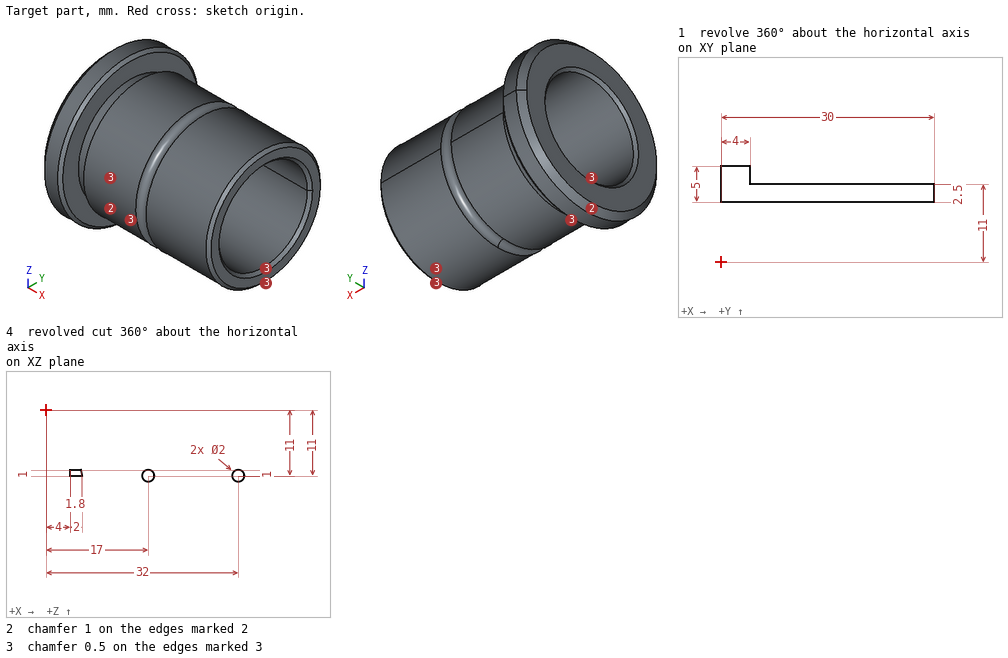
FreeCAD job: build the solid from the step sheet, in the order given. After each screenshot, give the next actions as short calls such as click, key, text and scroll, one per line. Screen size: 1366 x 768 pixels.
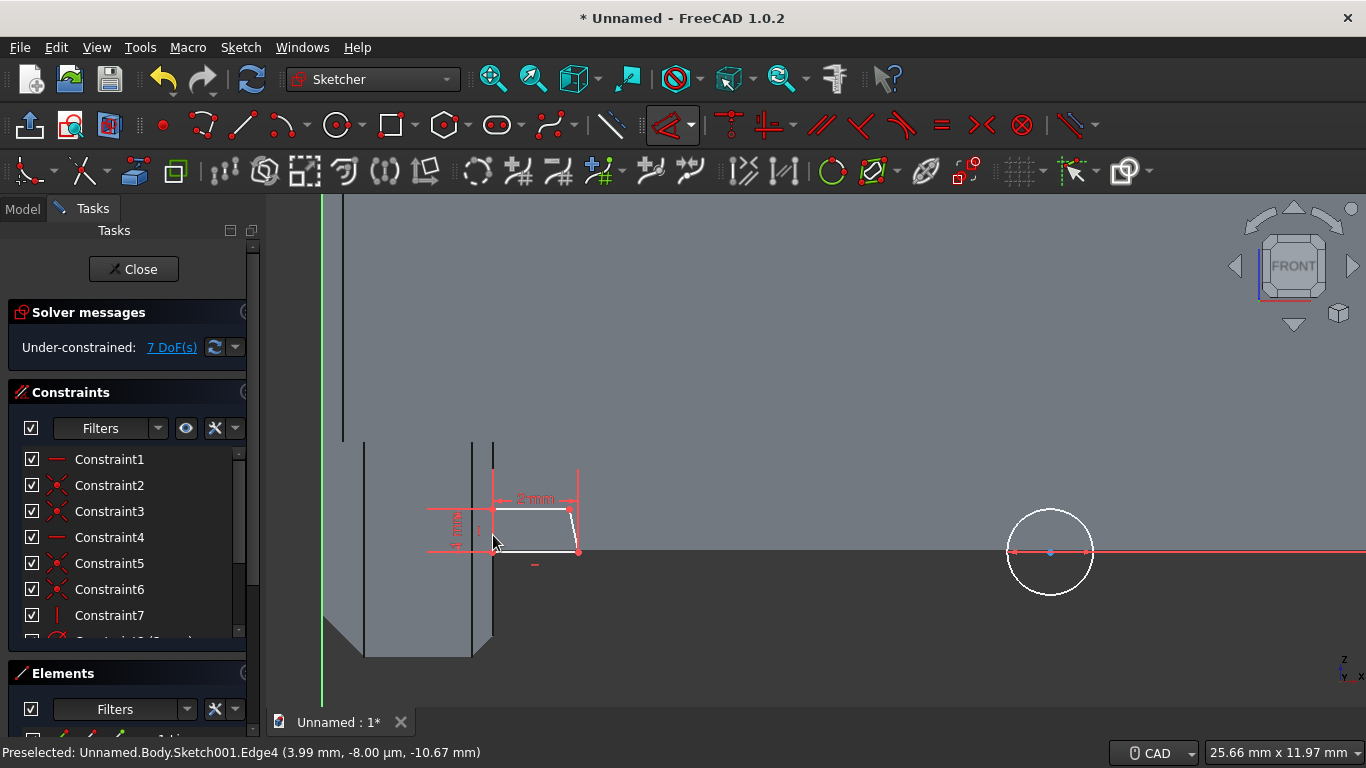
click(493, 509)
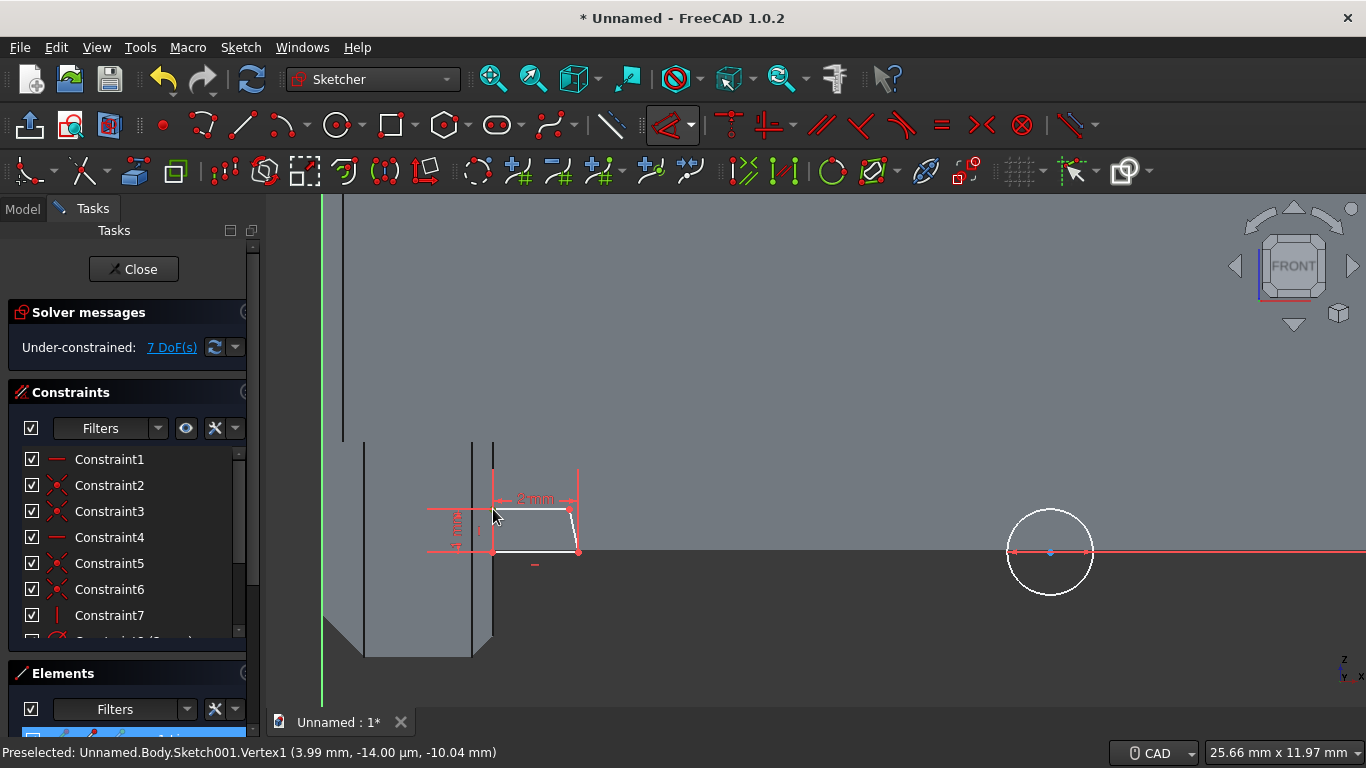
click(694, 126)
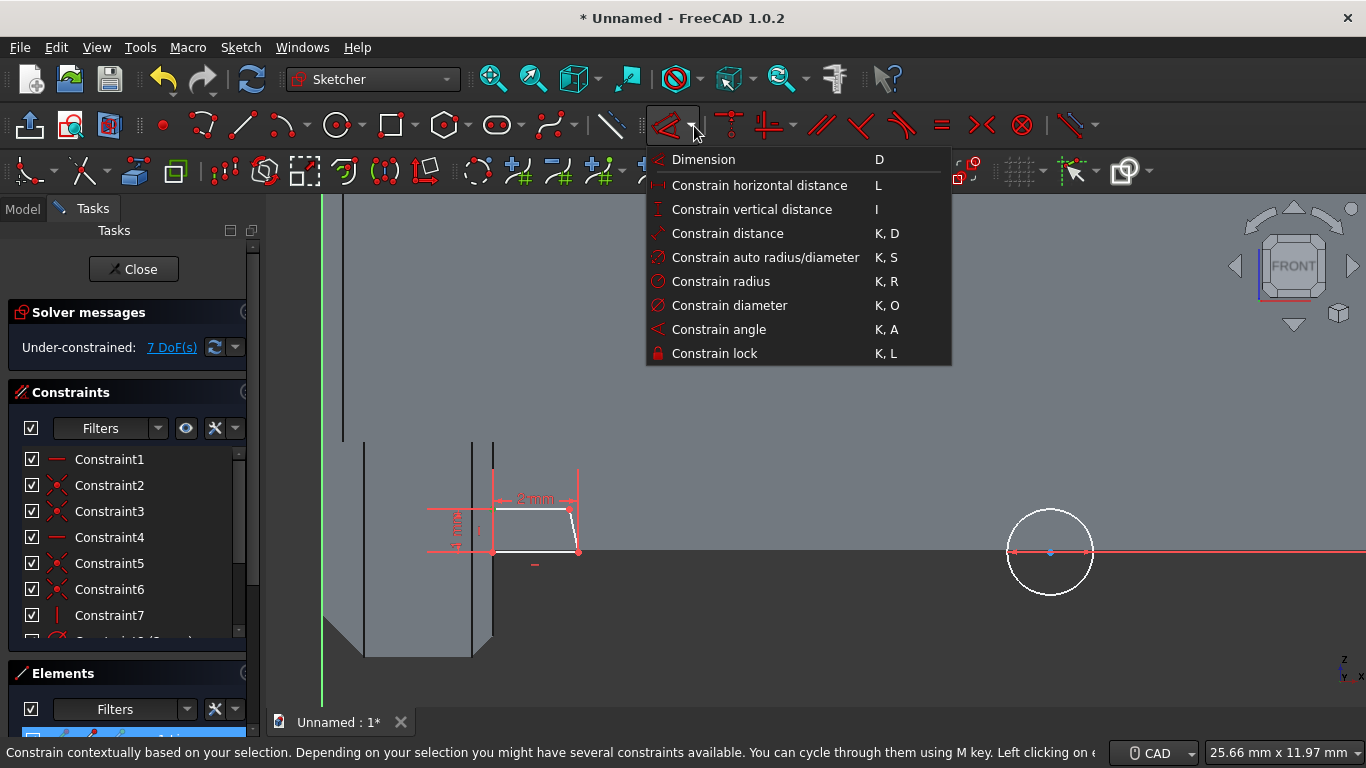
click(799, 185)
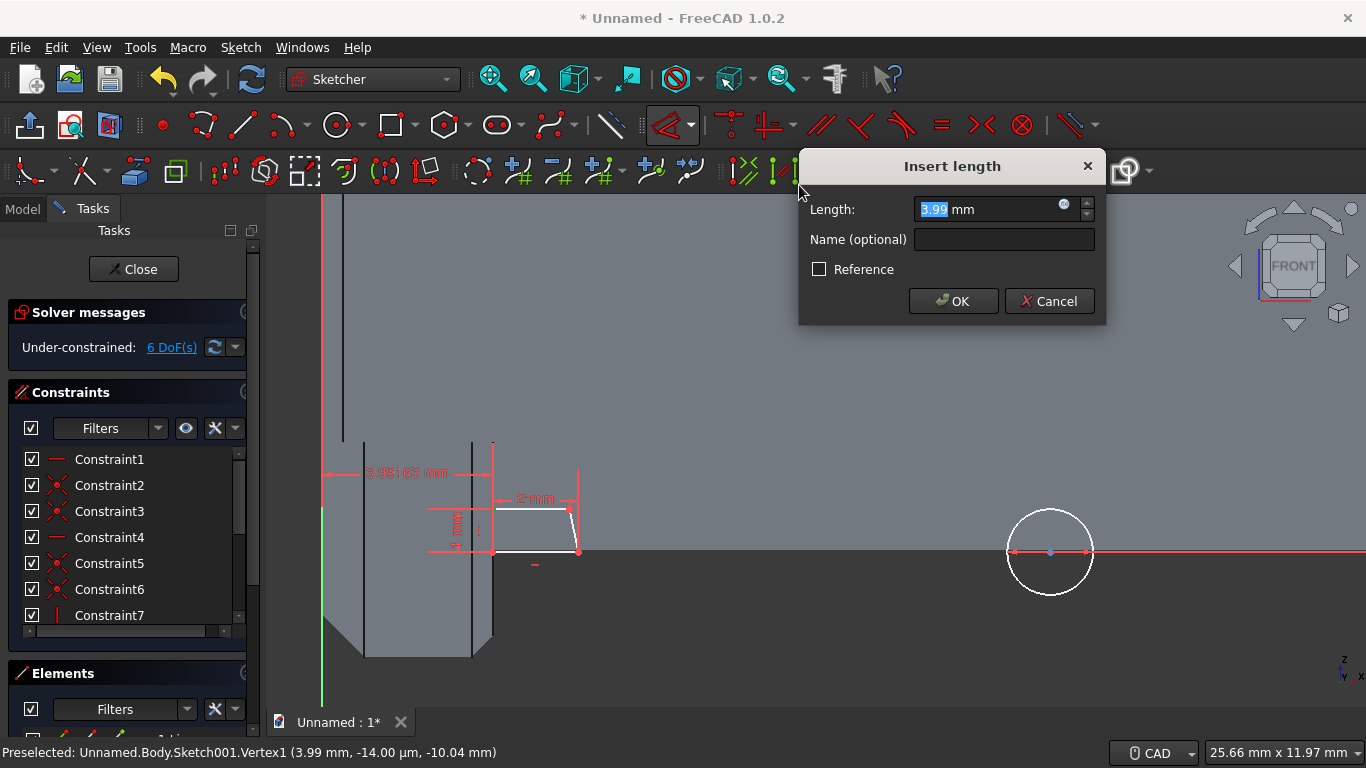
text(4)
key(Return)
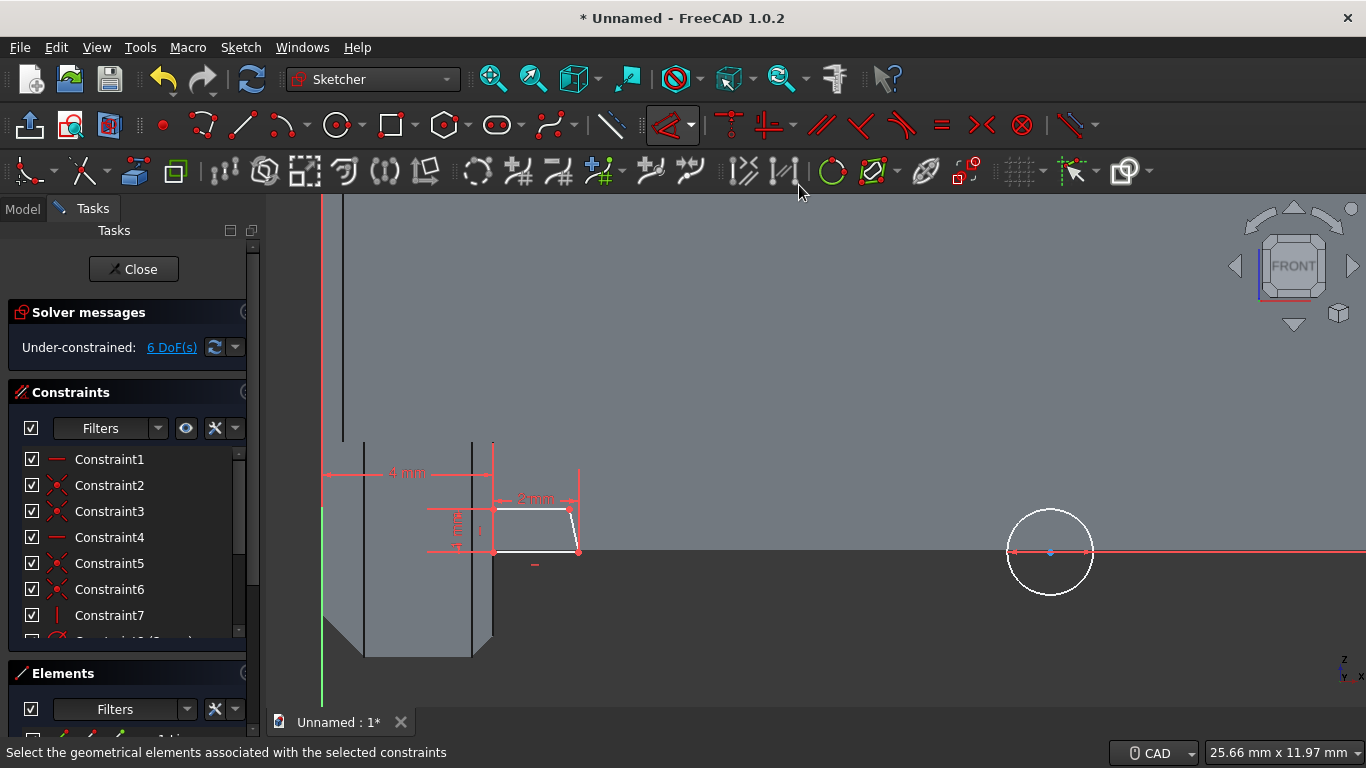
scroll(518, 544, down, 4)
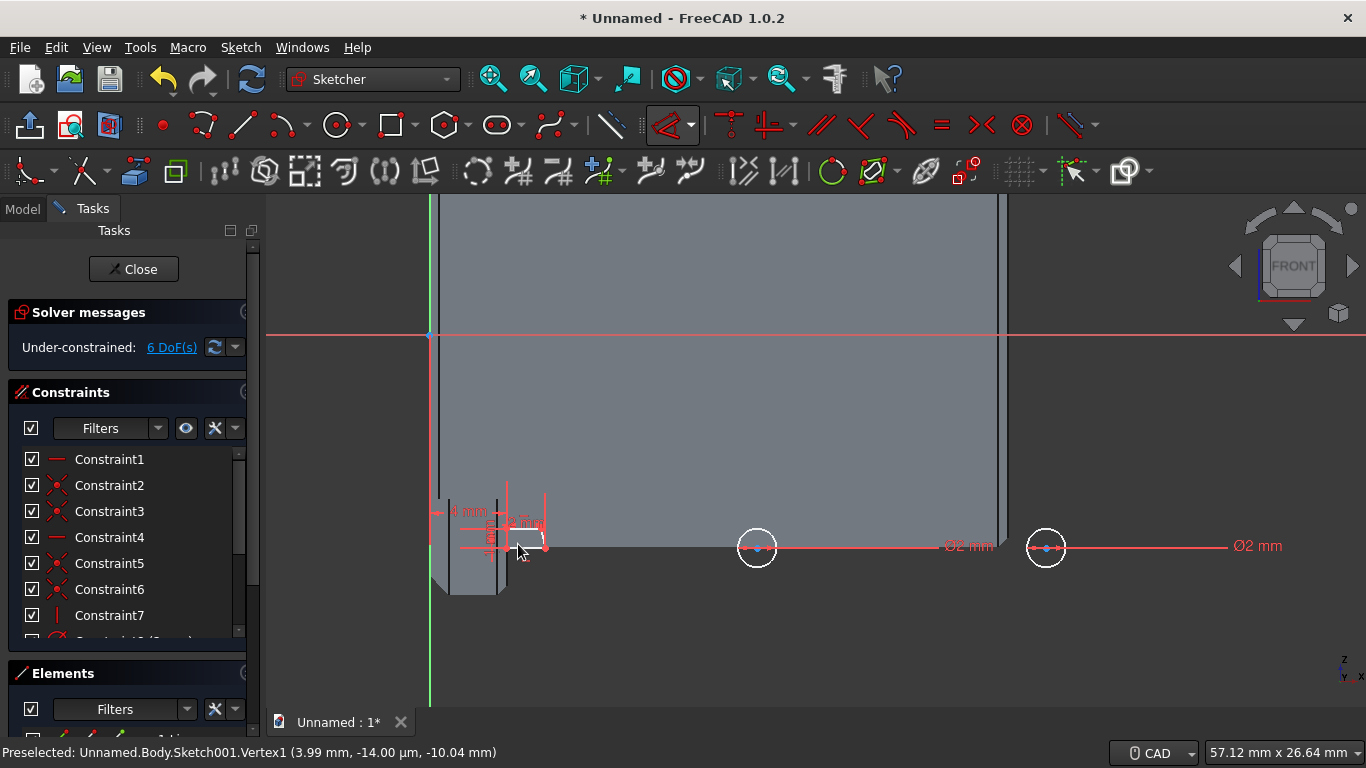
click(1046, 548)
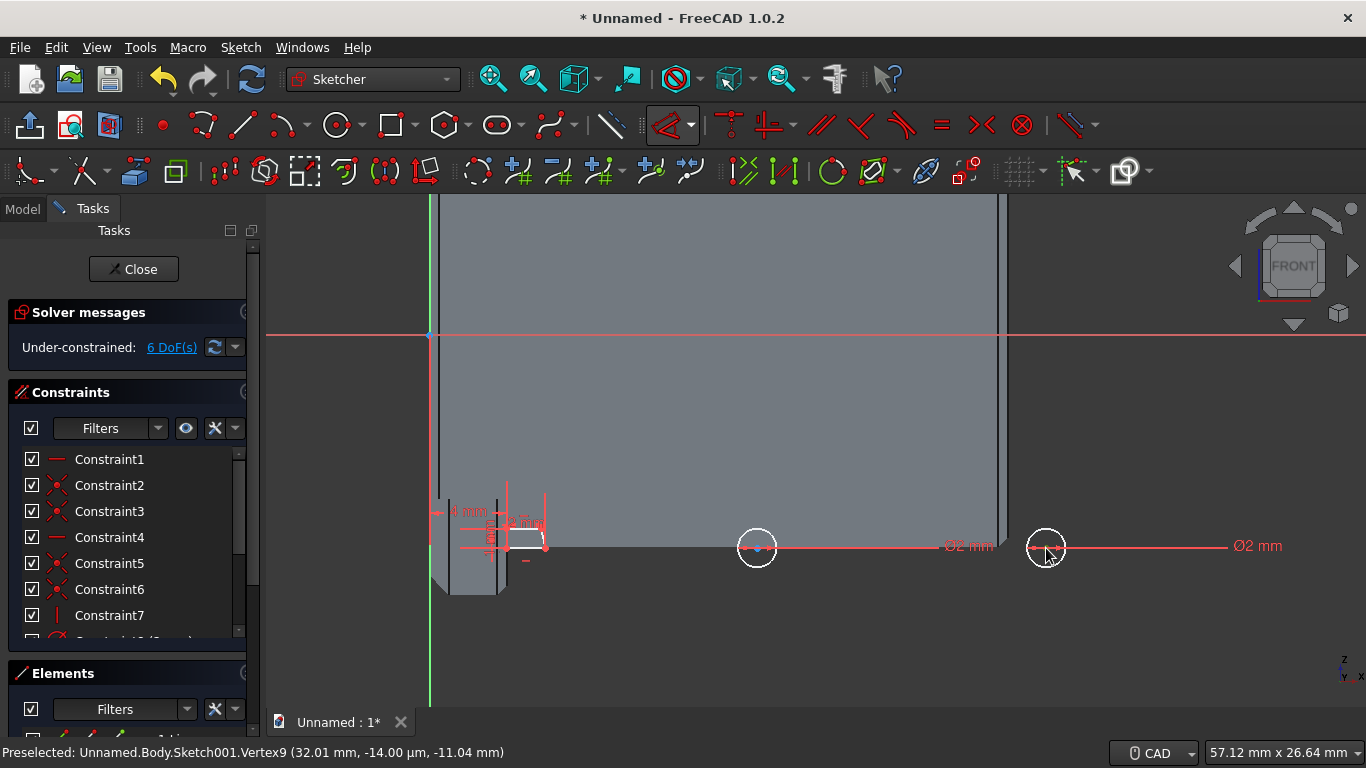
key(l)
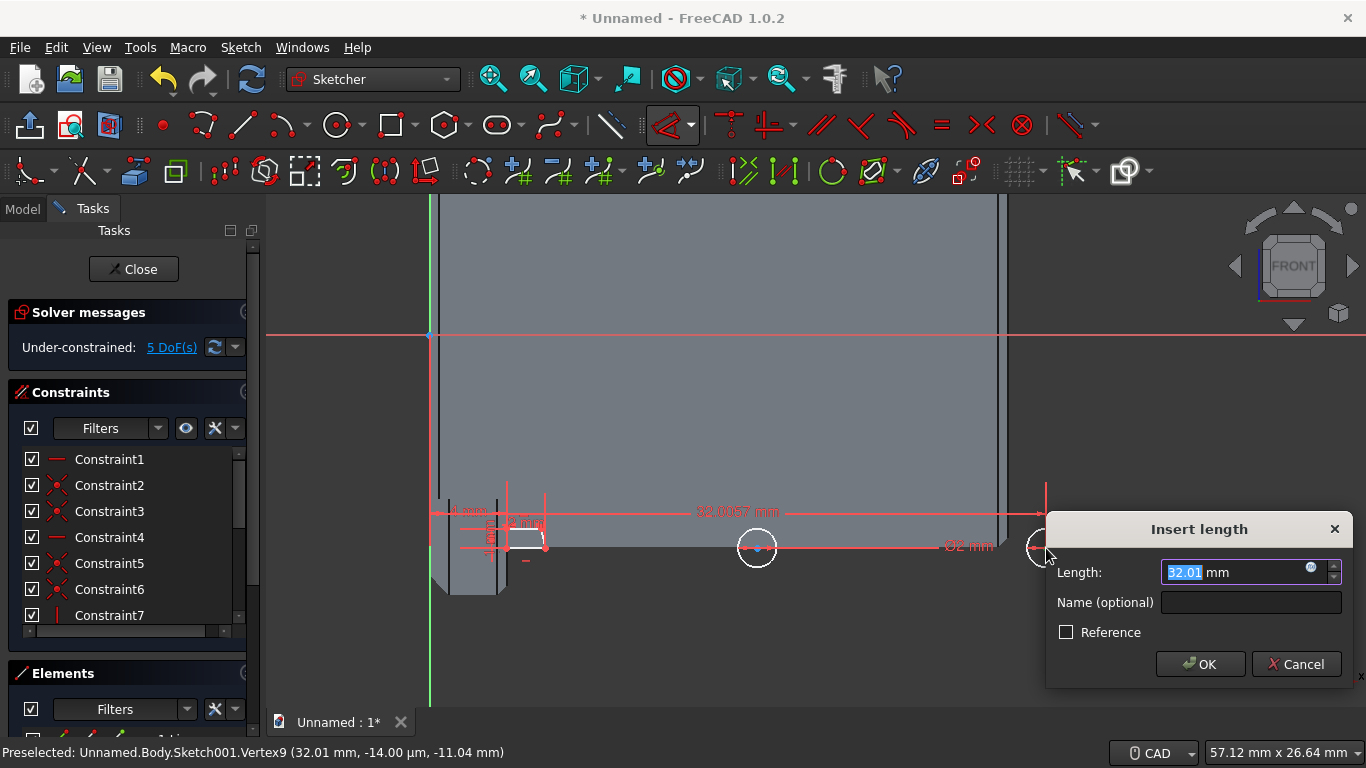
text(32)
key(Return)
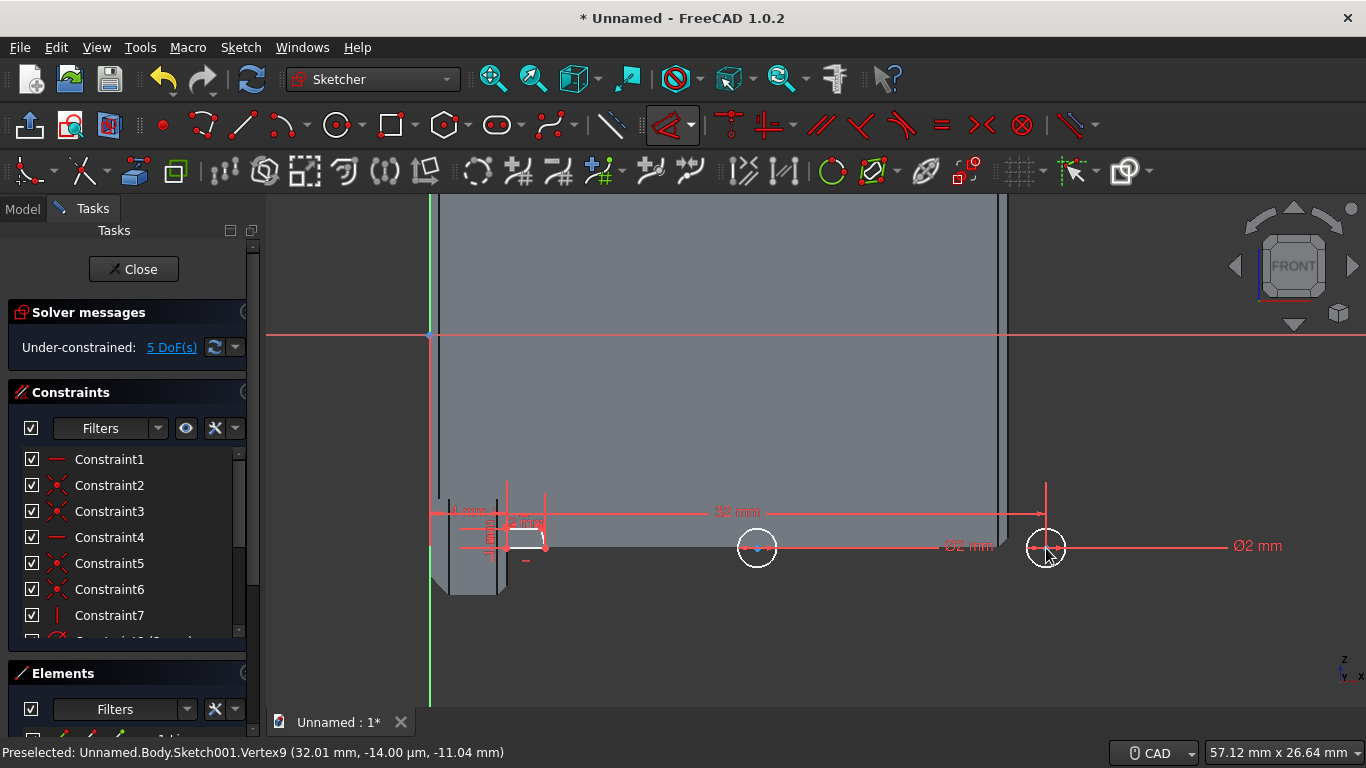
click(1046, 548)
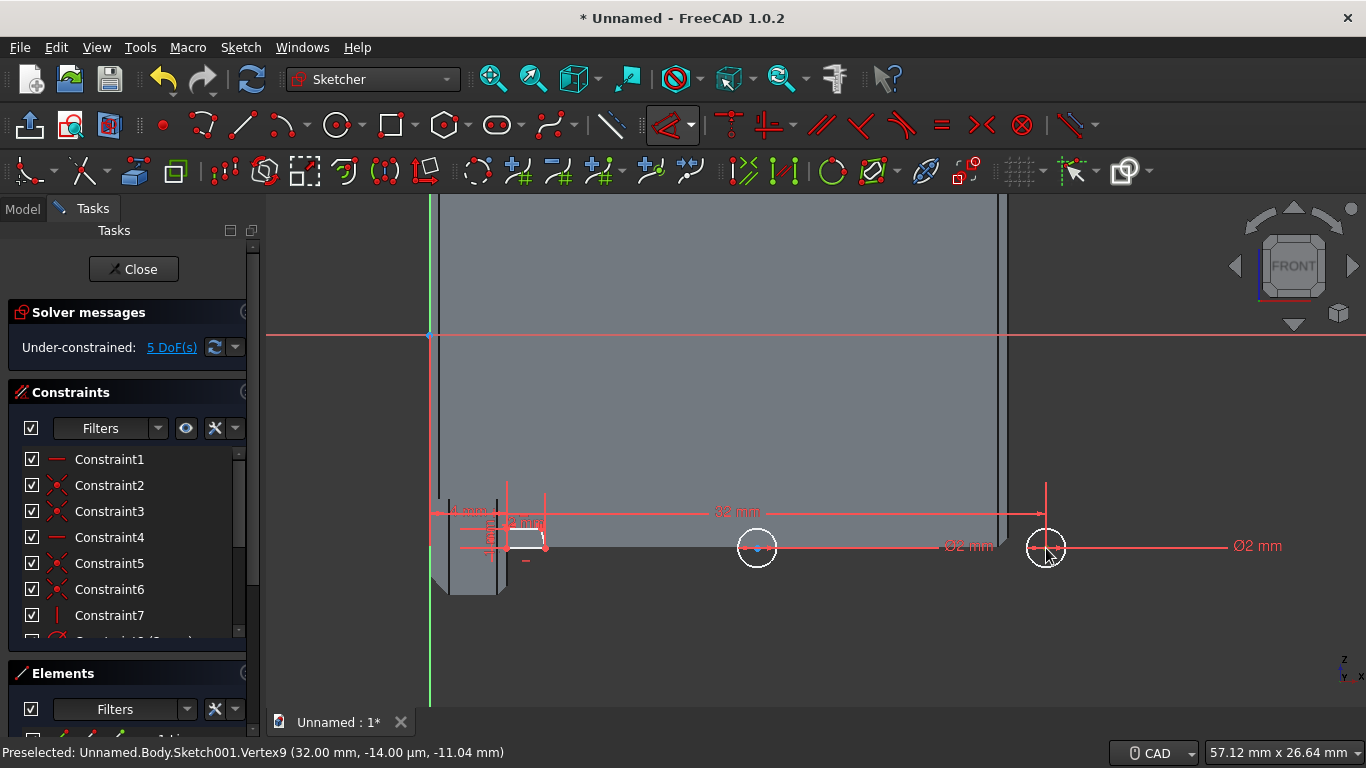
key(i)